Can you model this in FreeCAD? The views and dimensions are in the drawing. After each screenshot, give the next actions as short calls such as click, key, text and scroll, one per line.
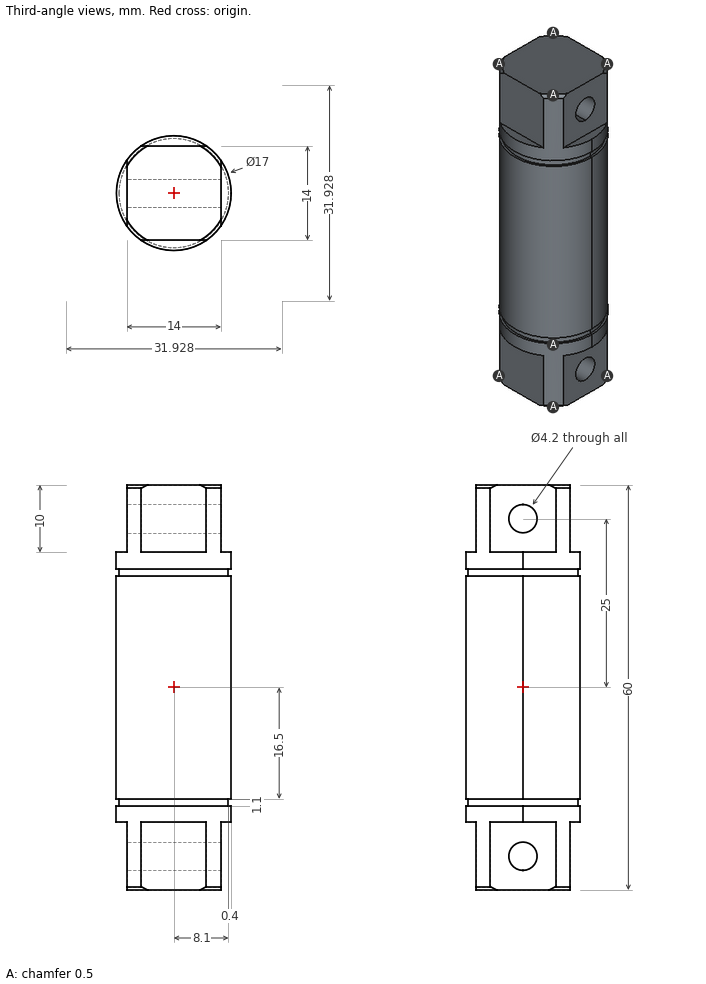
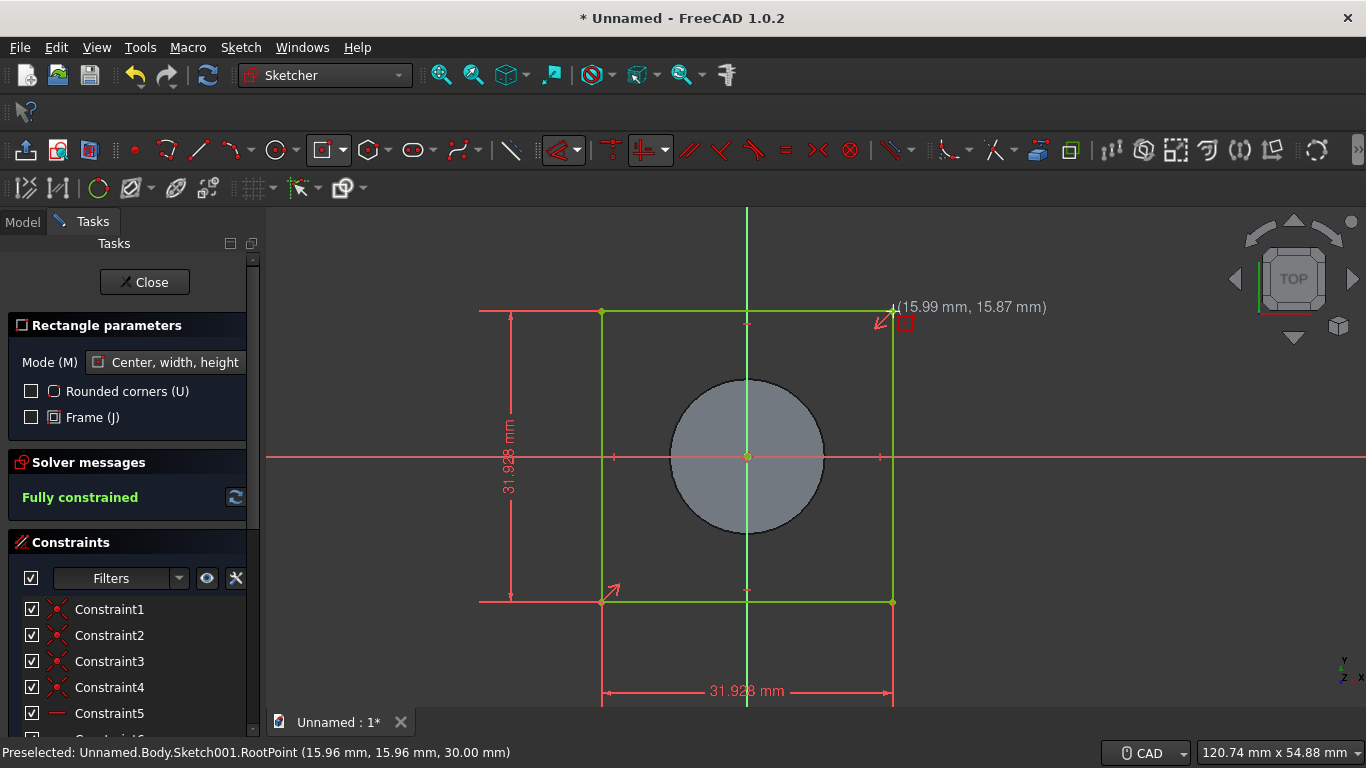
click(747, 457)
move(811, 393)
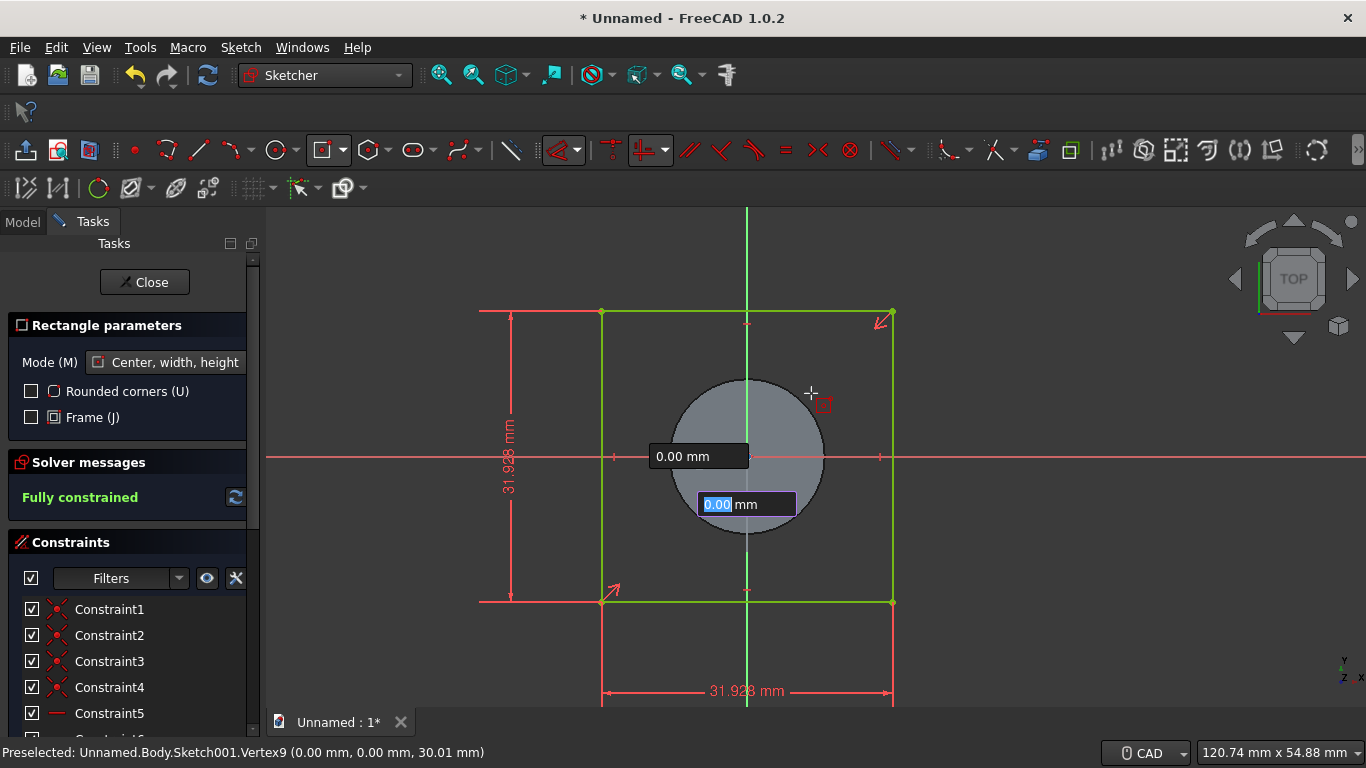
text(14)
key(Tab)
text(14)
key(Return)
key(Escape)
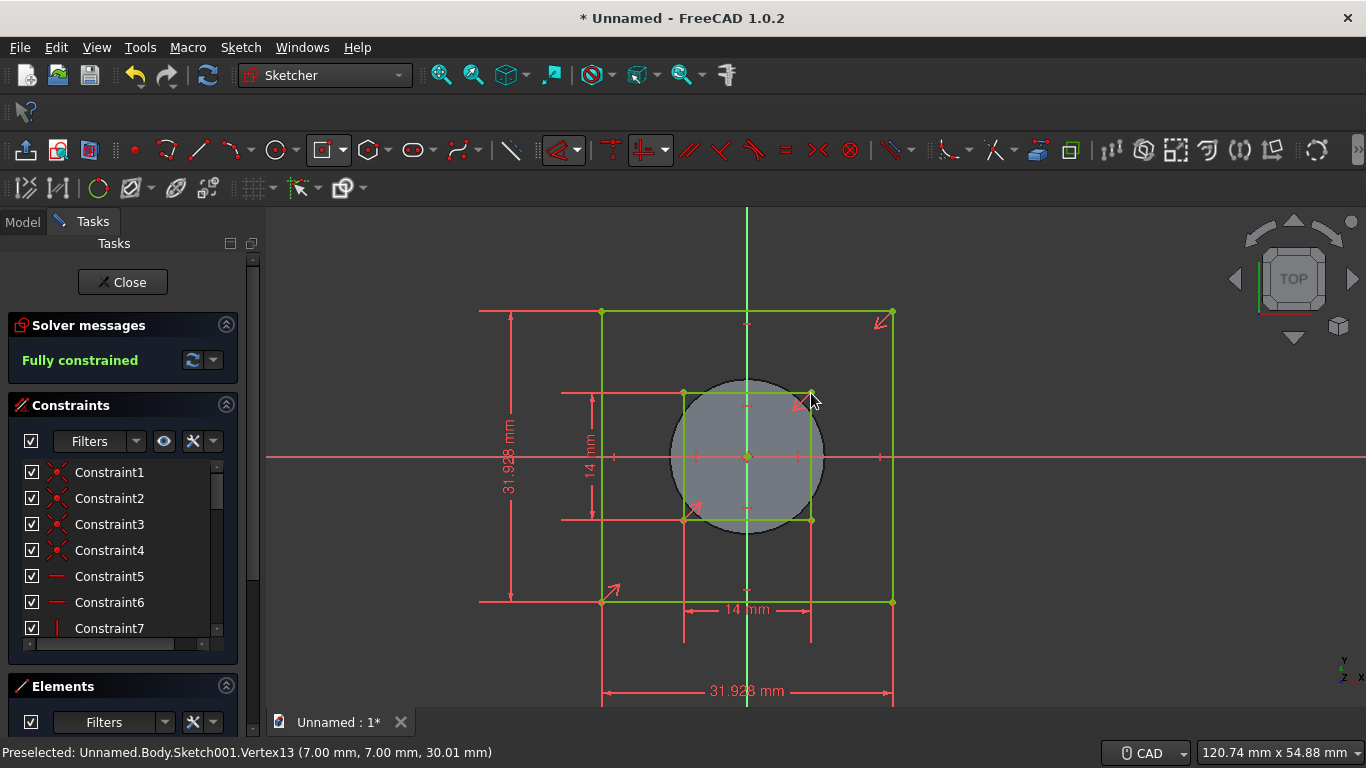
click(123, 282)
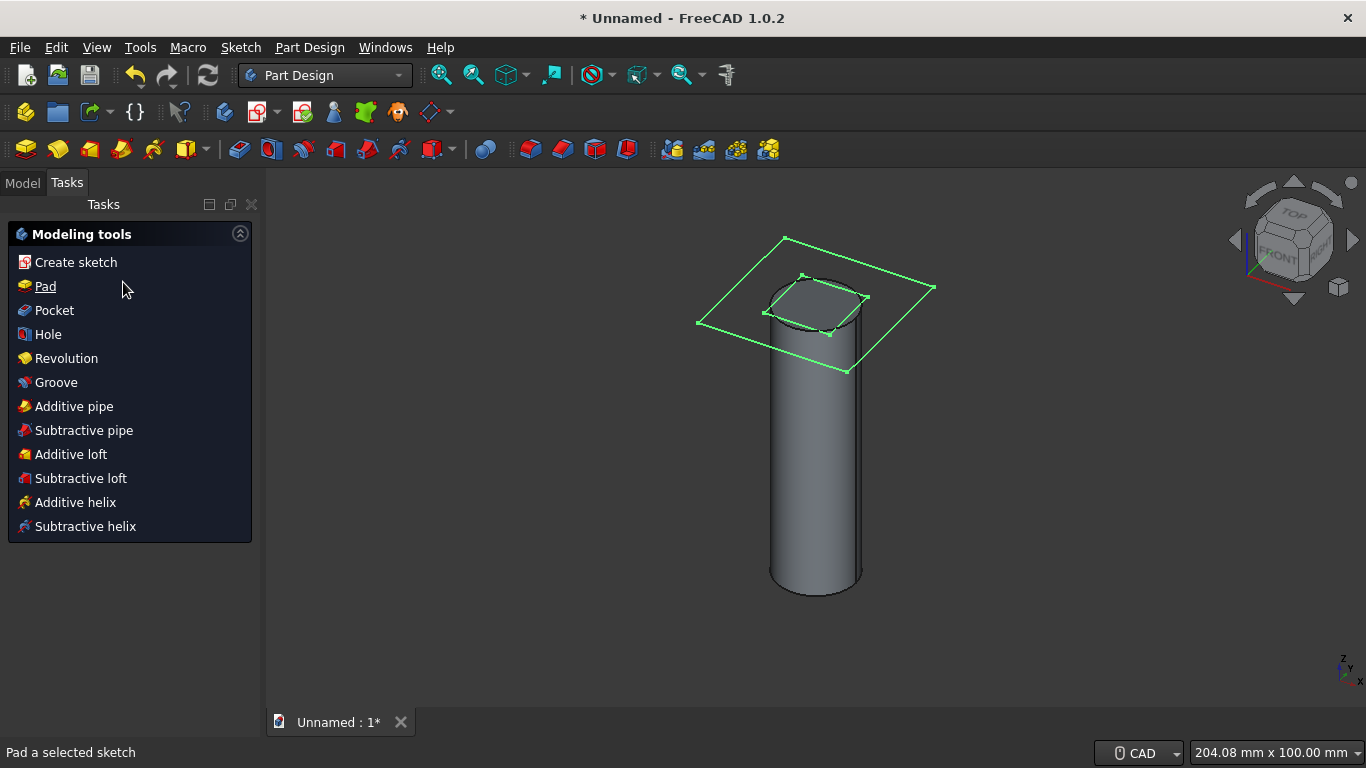
click(240, 150)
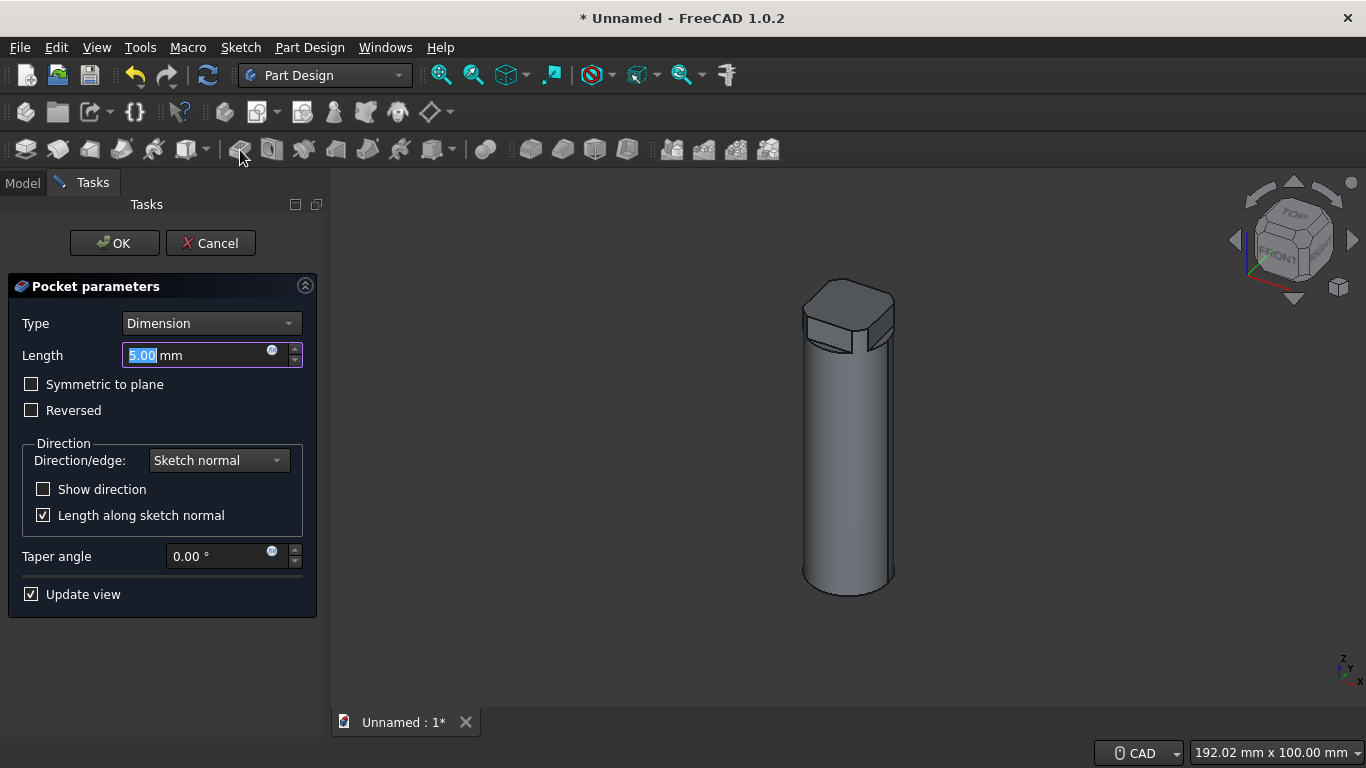
text(10)
key(Tab)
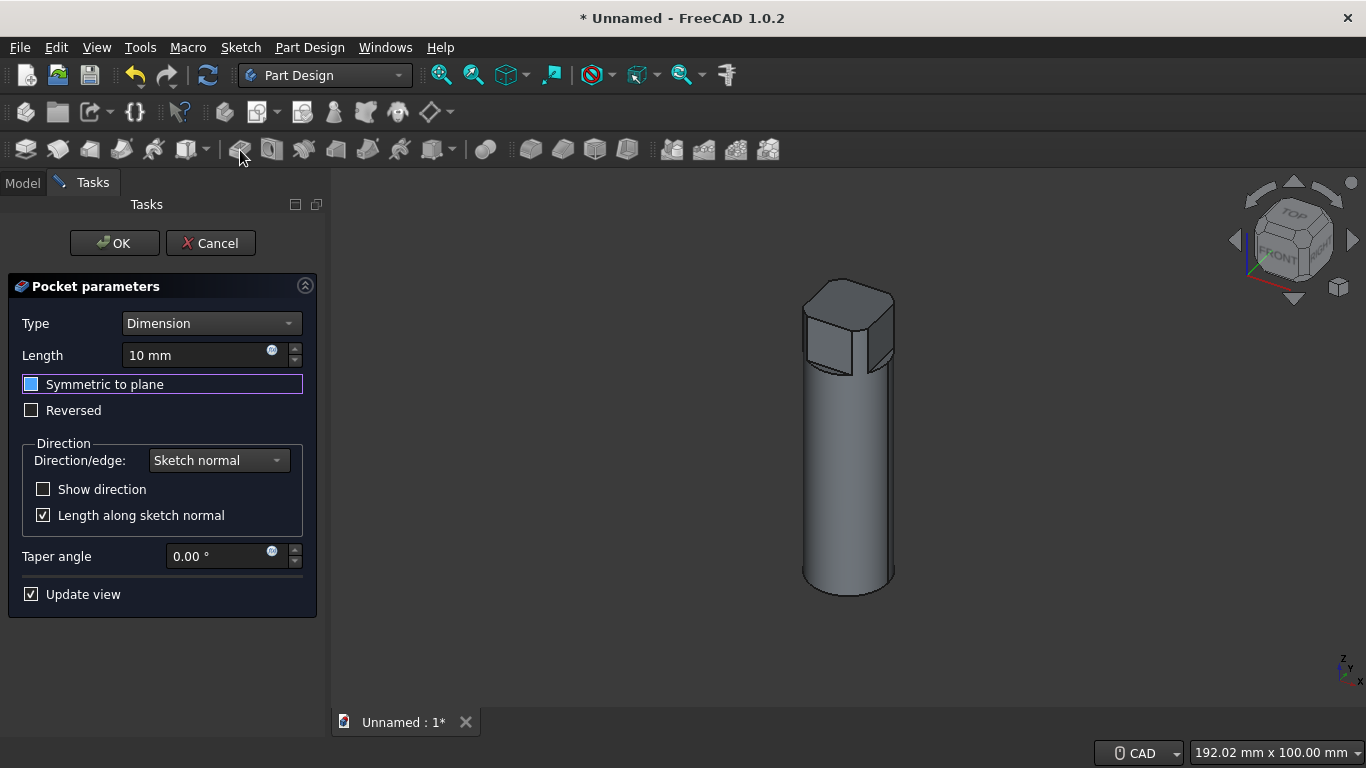
click(115, 243)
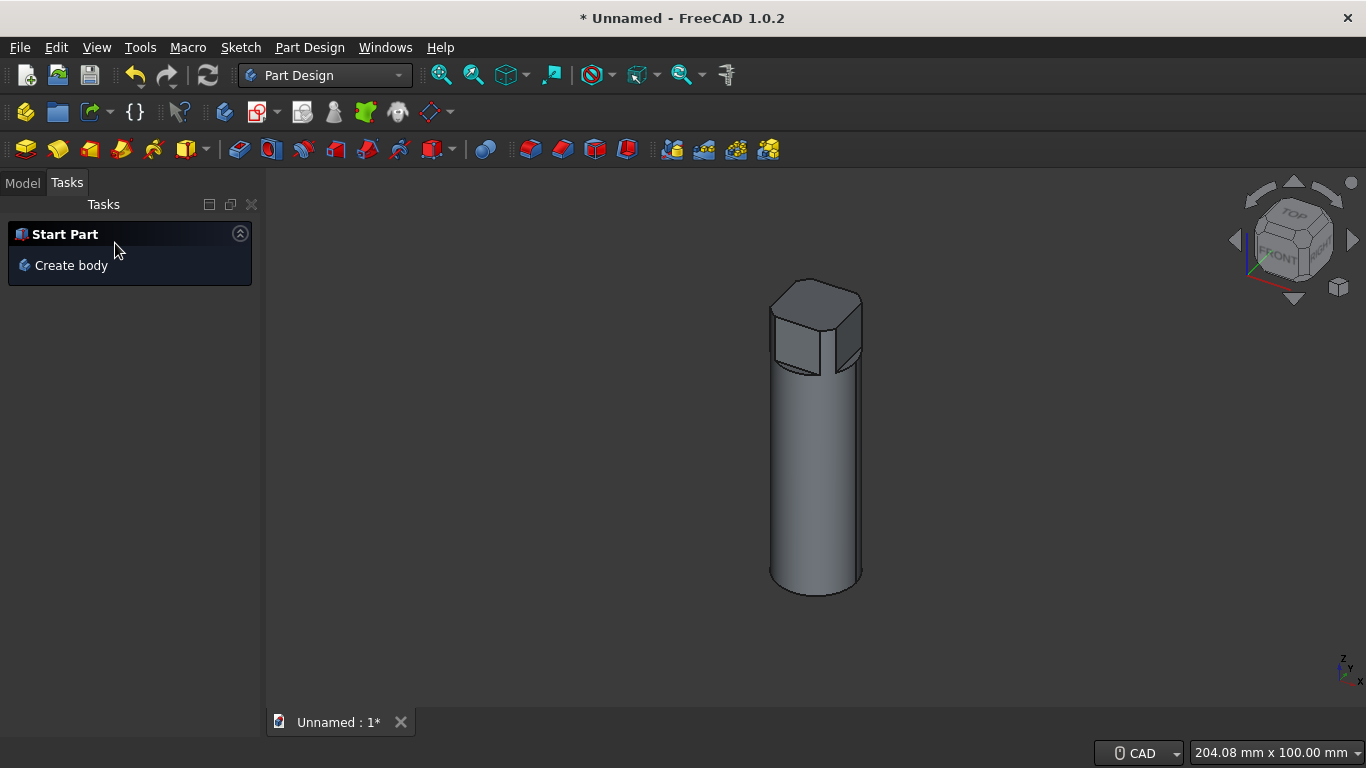
click(849, 337)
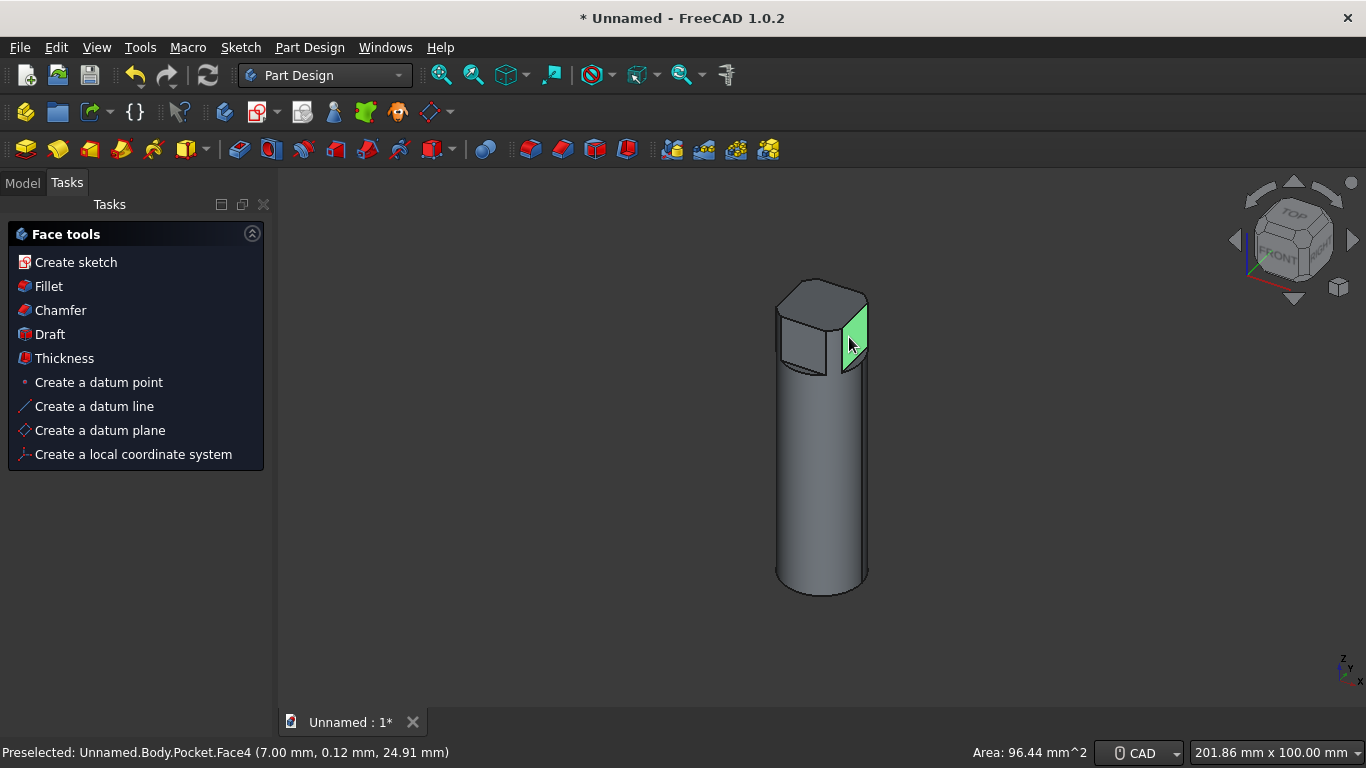
click(258, 112)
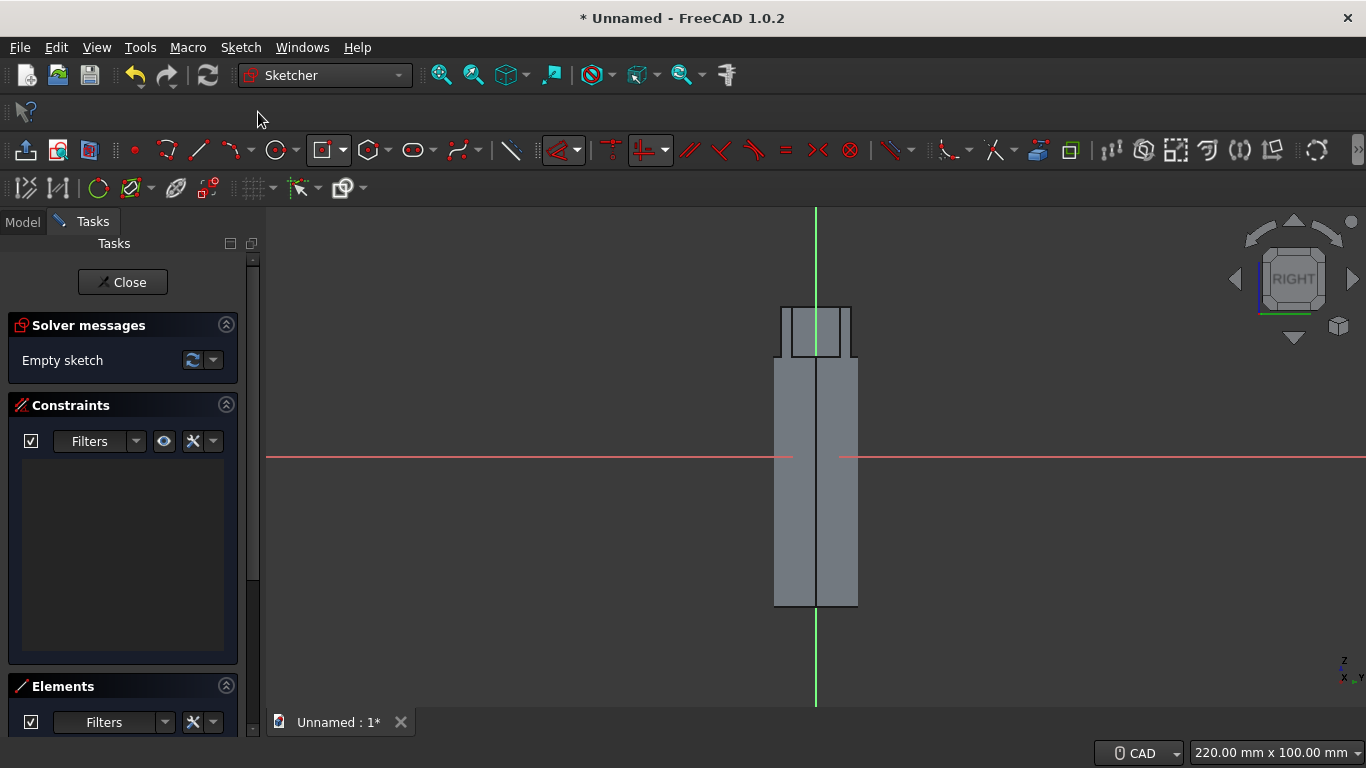
scroll(820, 324, up, 14)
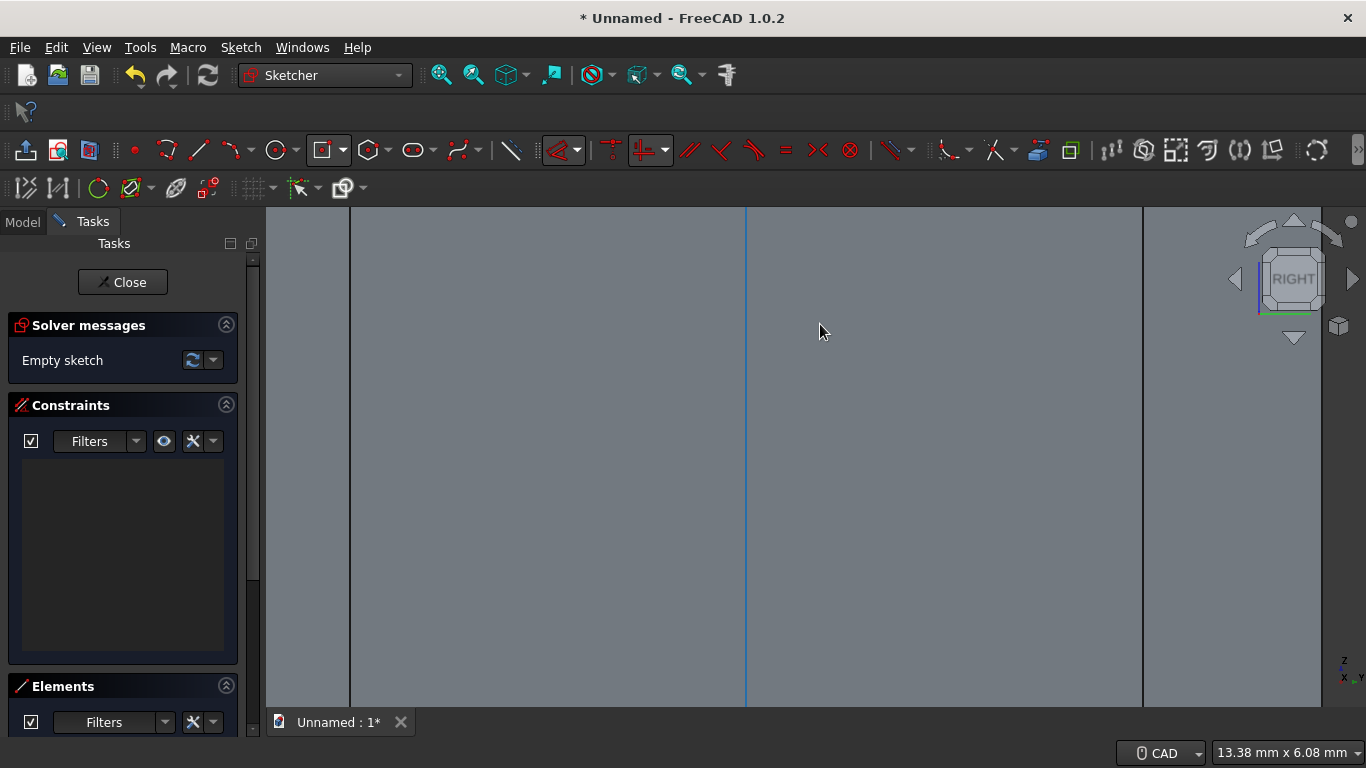
key(g)
key(c)